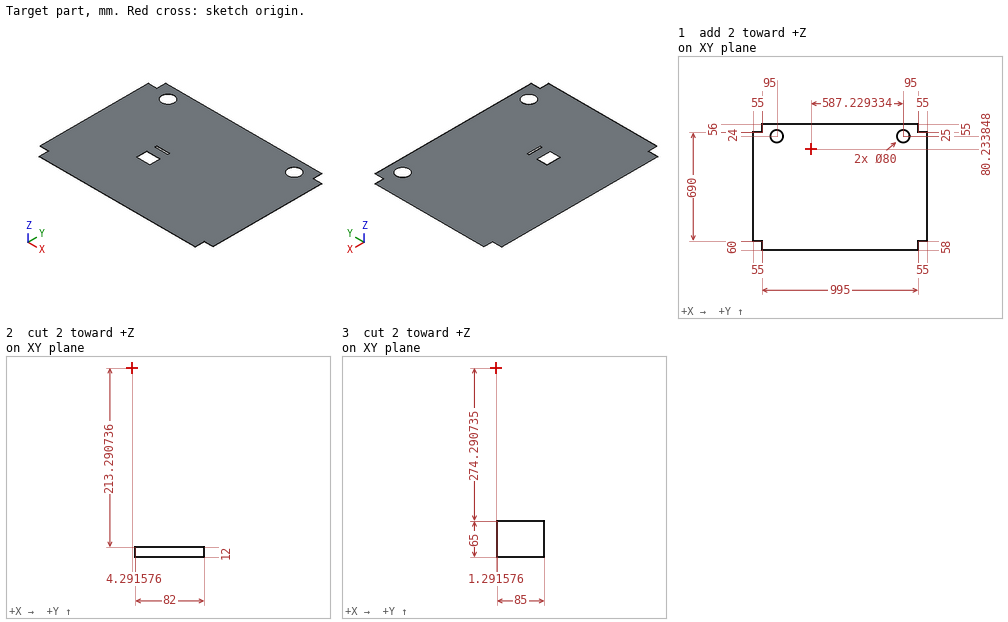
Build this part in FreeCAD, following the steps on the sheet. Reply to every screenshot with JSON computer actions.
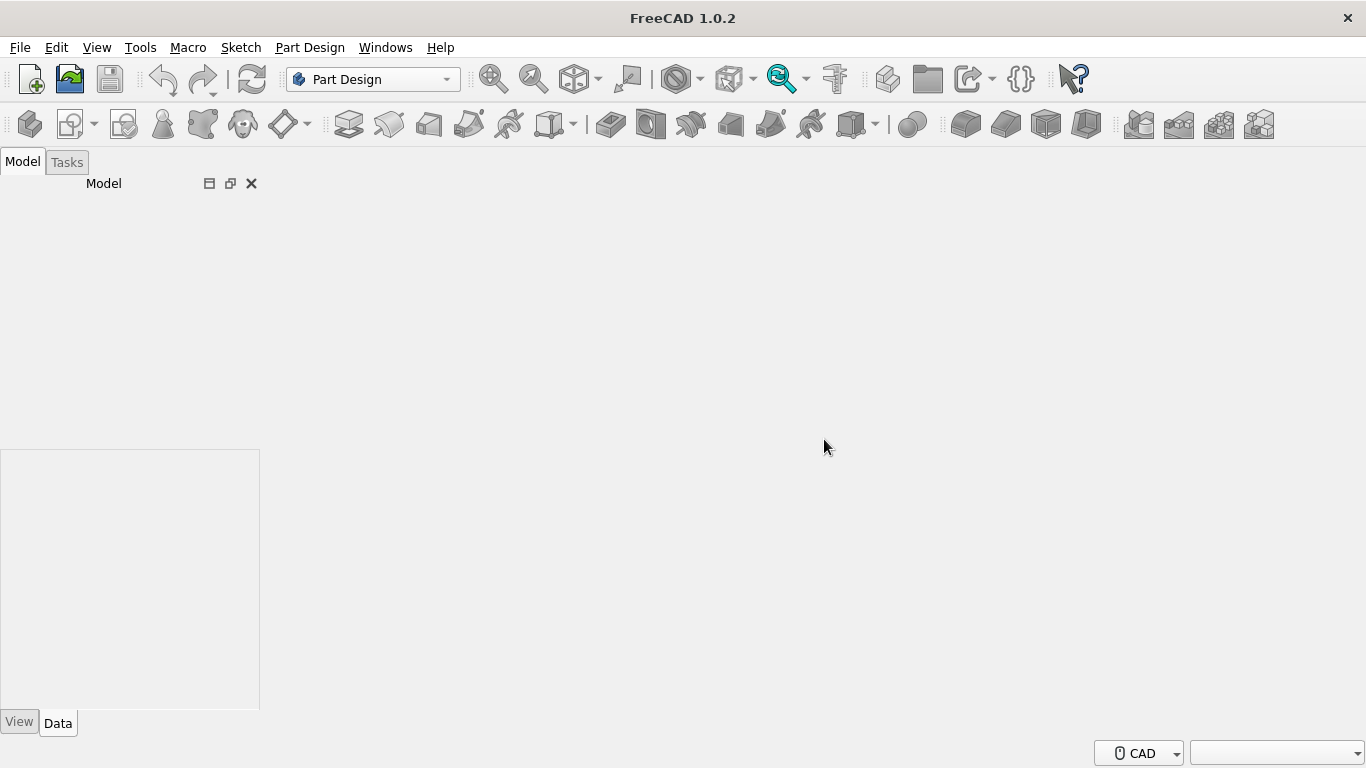
{"action": "left_click", "coordinate": [30, 80]}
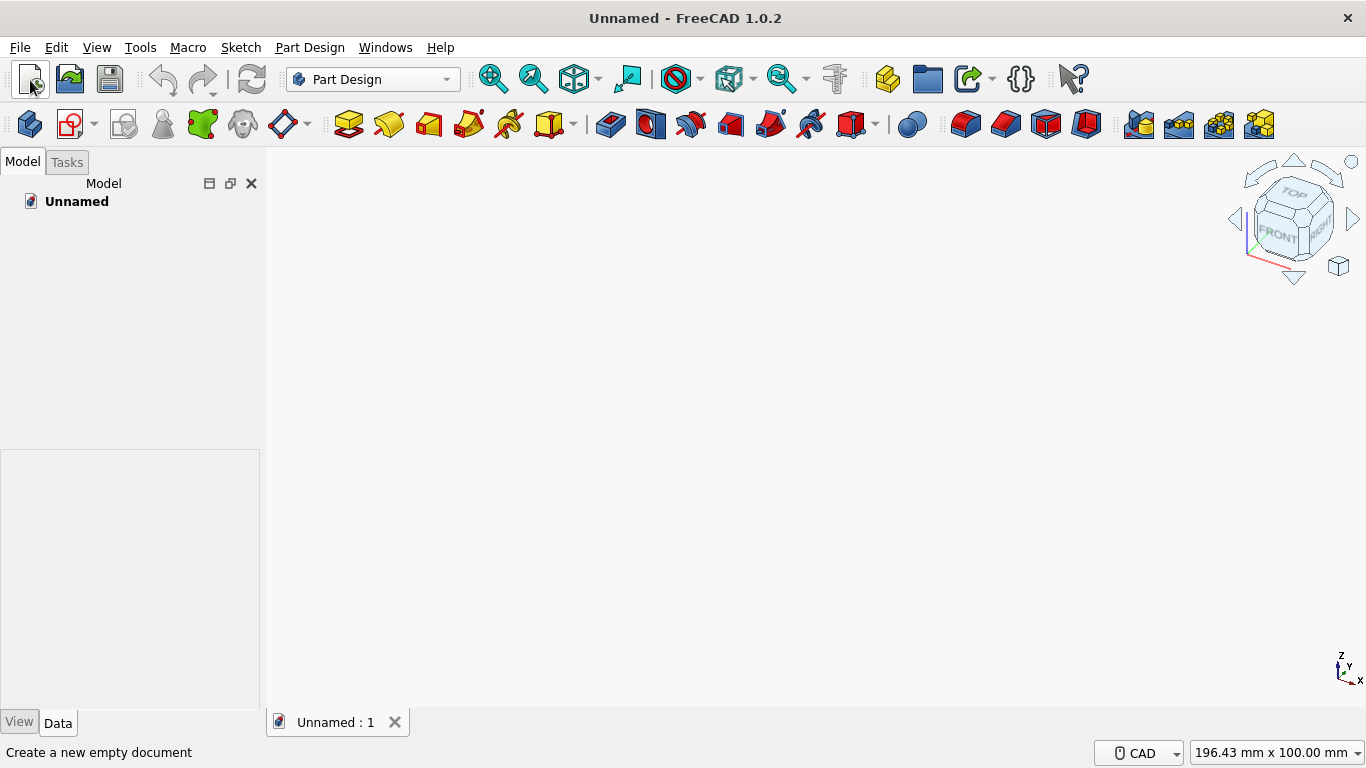
{"action": "left_click", "coordinate": [70, 124]}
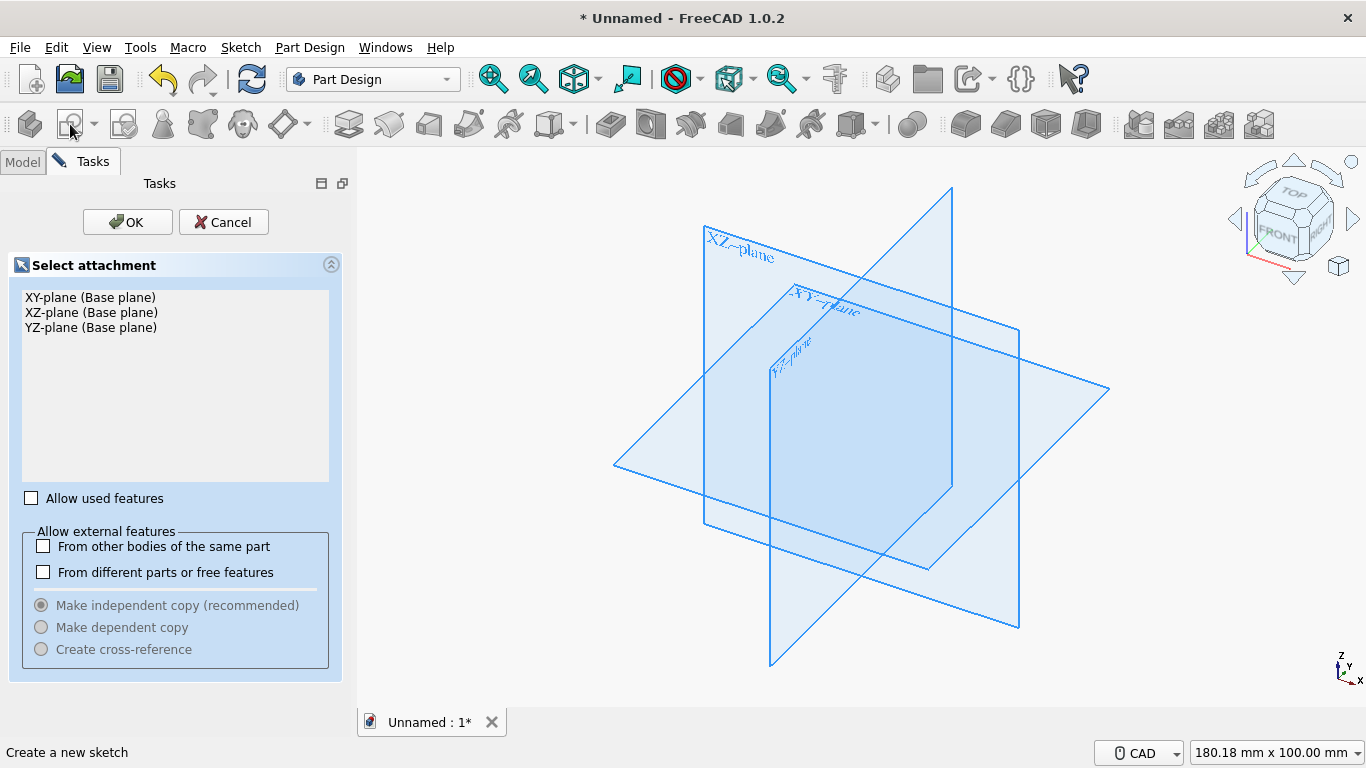
{"action": "left_click", "coordinate": [82, 298]}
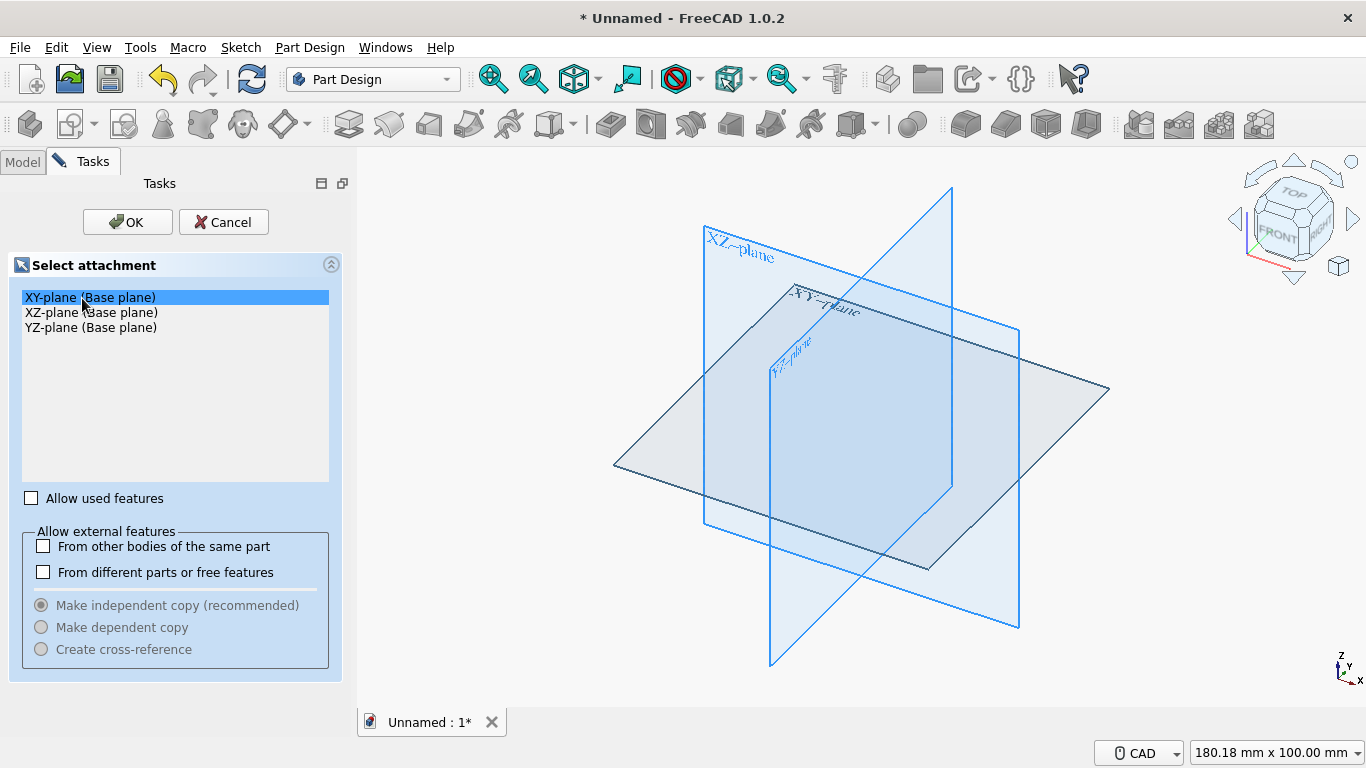
{"action": "left_click", "coordinate": [128, 222]}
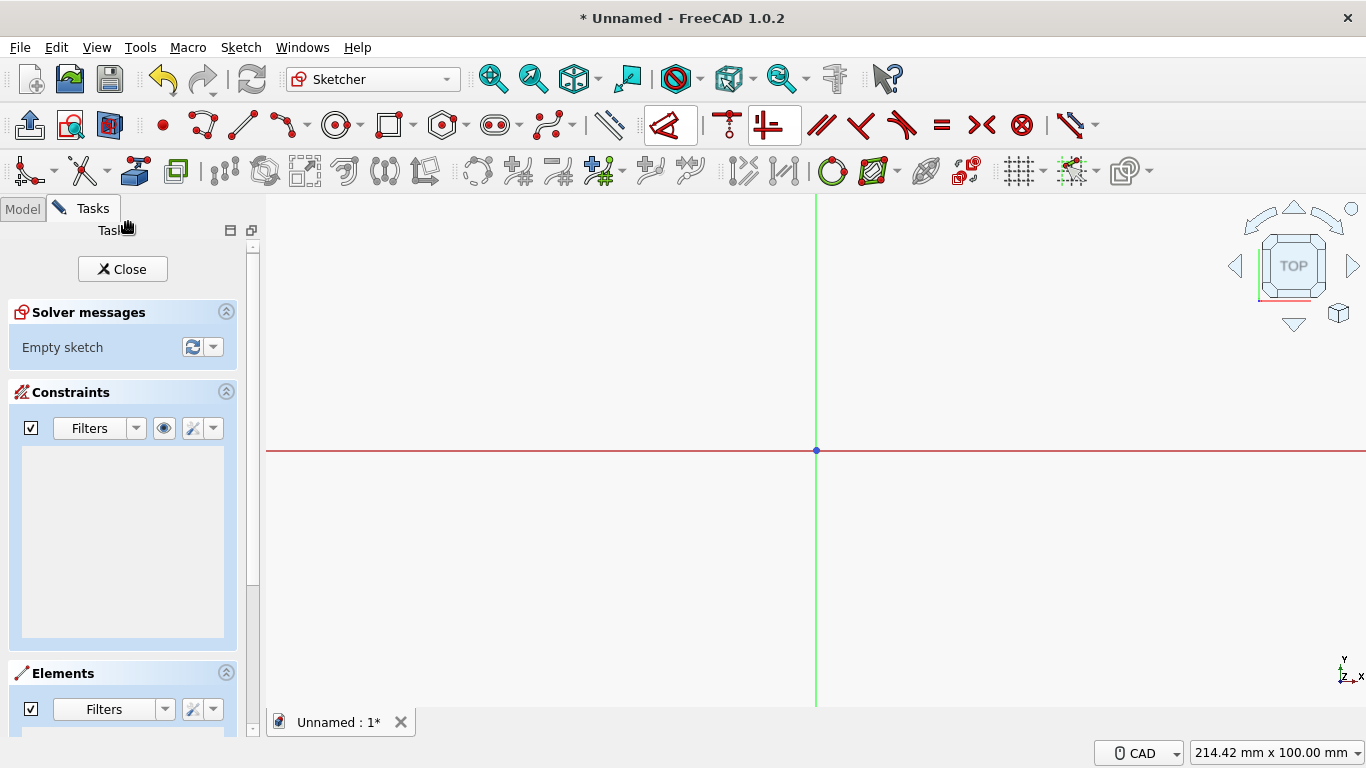
{"action": "scroll", "coordinate": [666, 351], "scroll_direction": "down", "scroll_amount": 13}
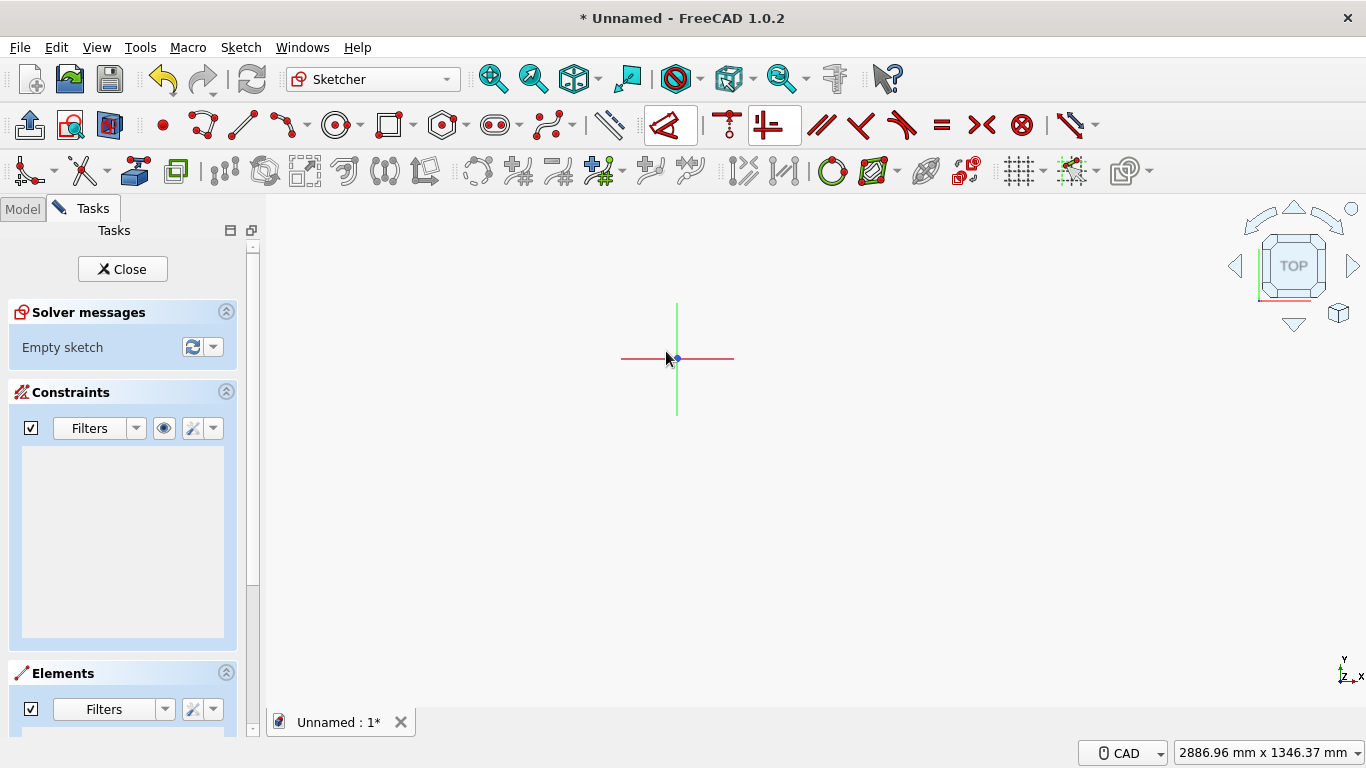
{"action": "left_click", "coordinate": [204, 126]}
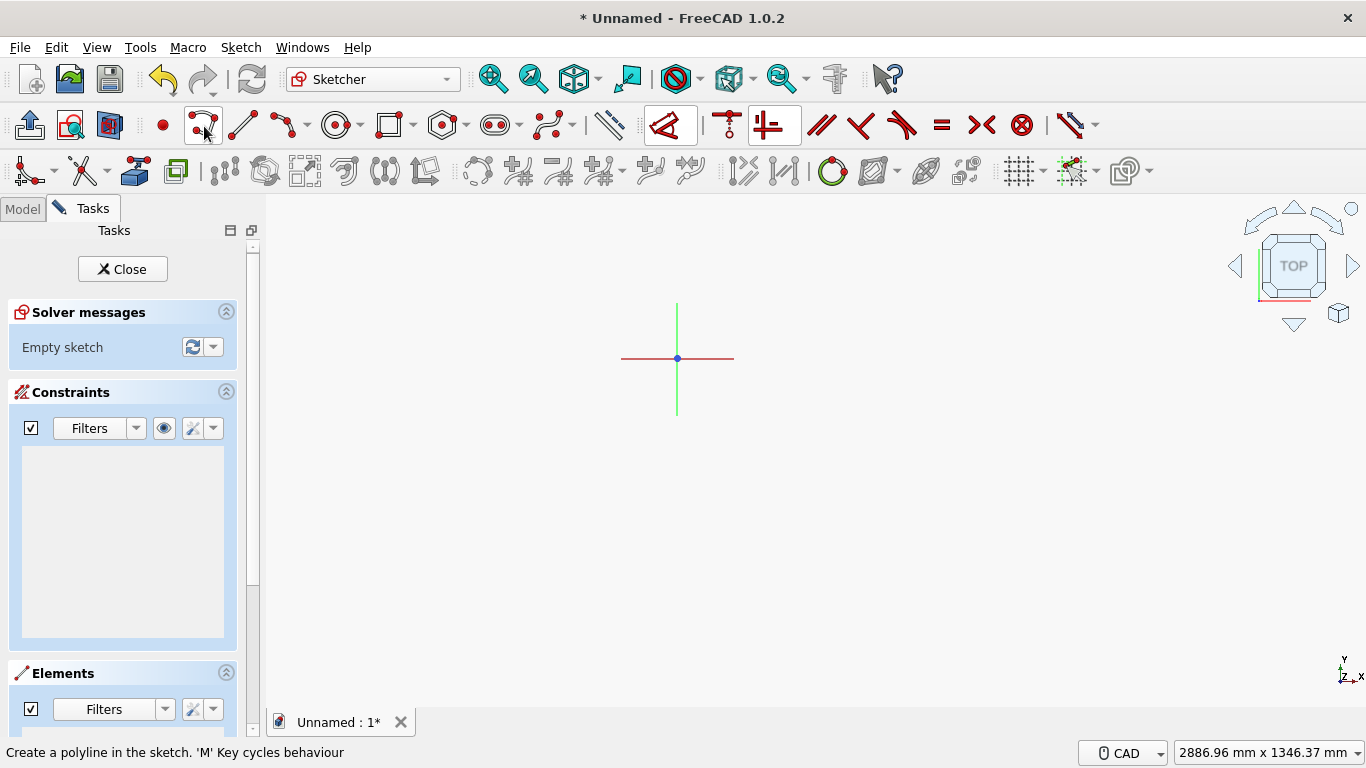
{"action": "left_click", "coordinate": [558, 319]}
{"action": "left_click", "coordinate": [537, 319]}
{"action": "left_click", "coordinate": [537, 582]}
{"action": "left_click", "coordinate": [558, 582]}
{"action": "left_click", "coordinate": [558, 605]}
{"action": "left_click", "coordinate": [937, 605]}
{"action": "left_click", "coordinate": [937, 583]}
{"action": "left_click", "coordinate": [958, 583]}
{"action": "left_click", "coordinate": [958, 319]}
{"action": "left_click", "coordinate": [937, 319]}
{"action": "left_click", "coordinate": [937, 298]}
{"action": "left_click", "coordinate": [558, 298]}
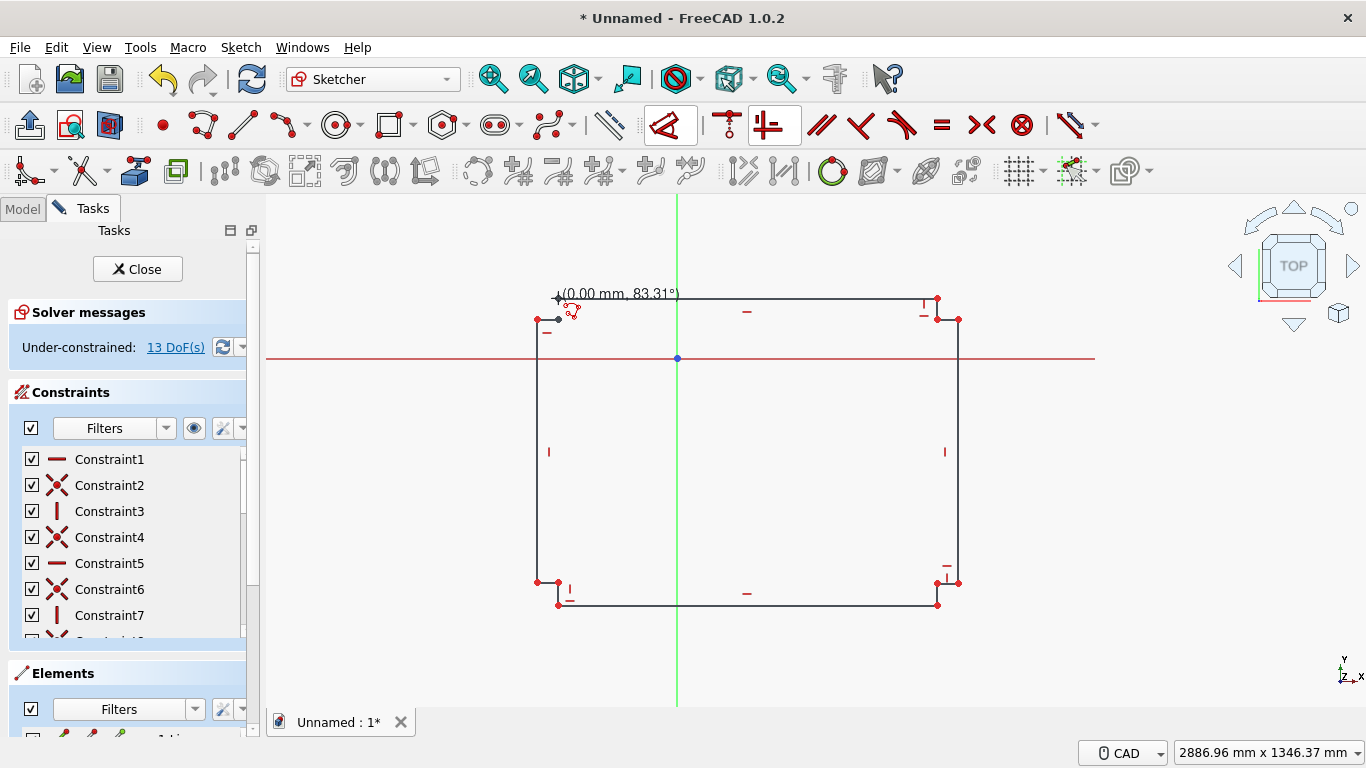
{"action": "scroll", "coordinate": [558, 319], "scroll_direction": "up", "scroll_amount": 3}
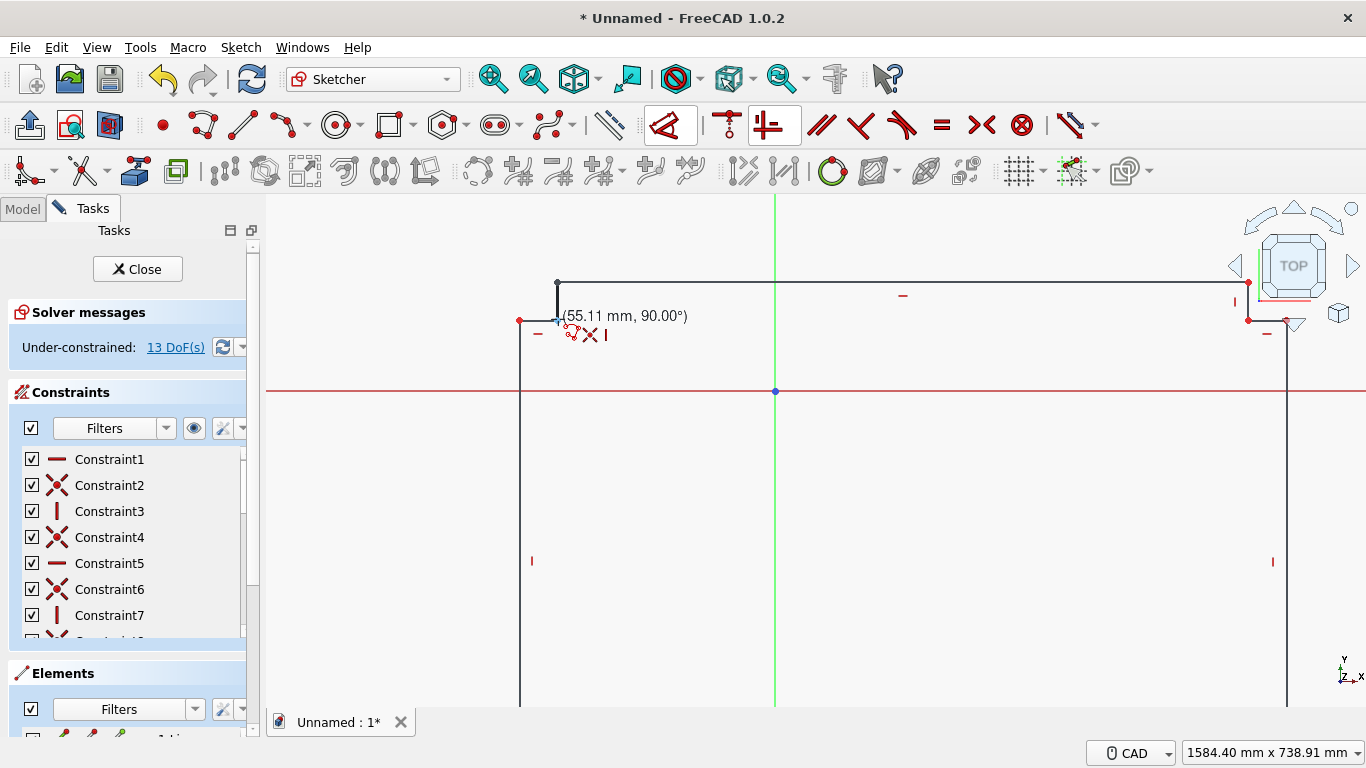
{"action": "left_click", "coordinate": [558, 321]}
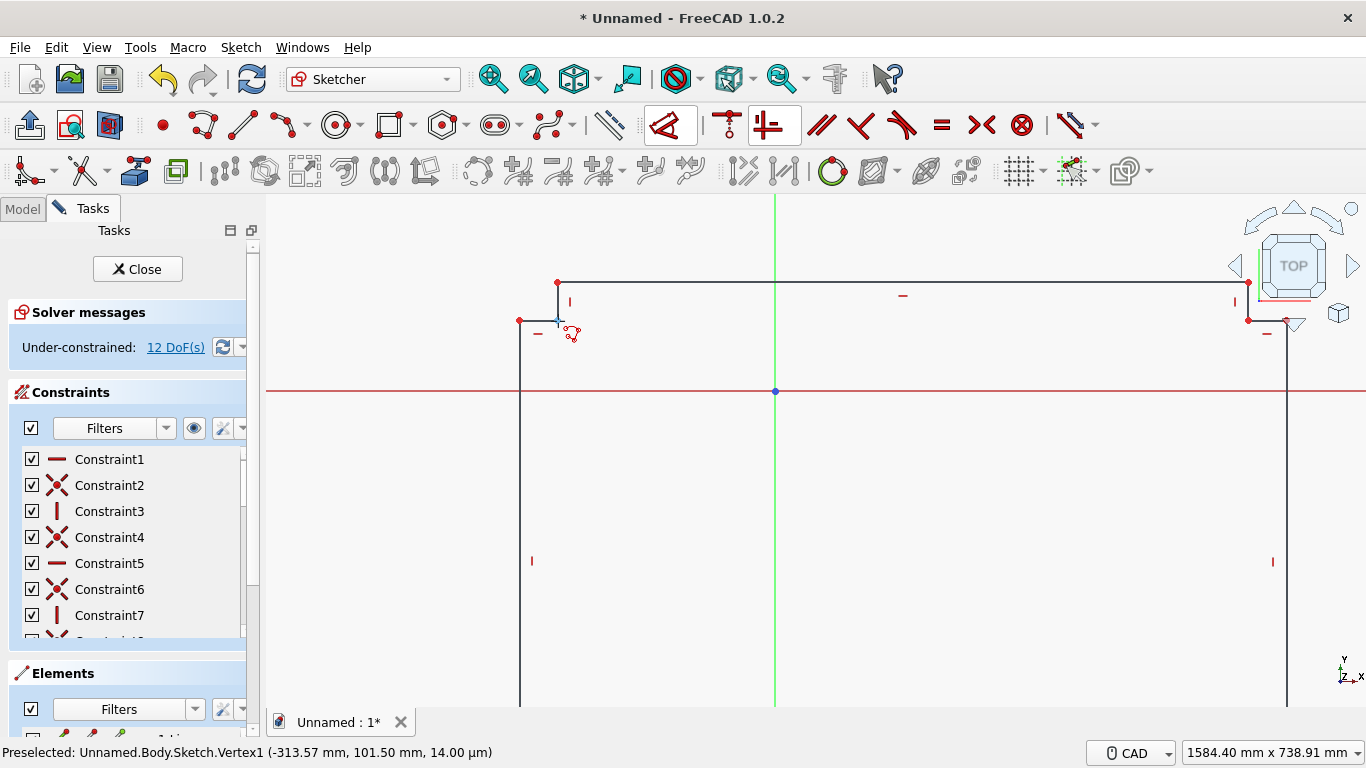
{"action": "left_click", "coordinate": [336, 126]}